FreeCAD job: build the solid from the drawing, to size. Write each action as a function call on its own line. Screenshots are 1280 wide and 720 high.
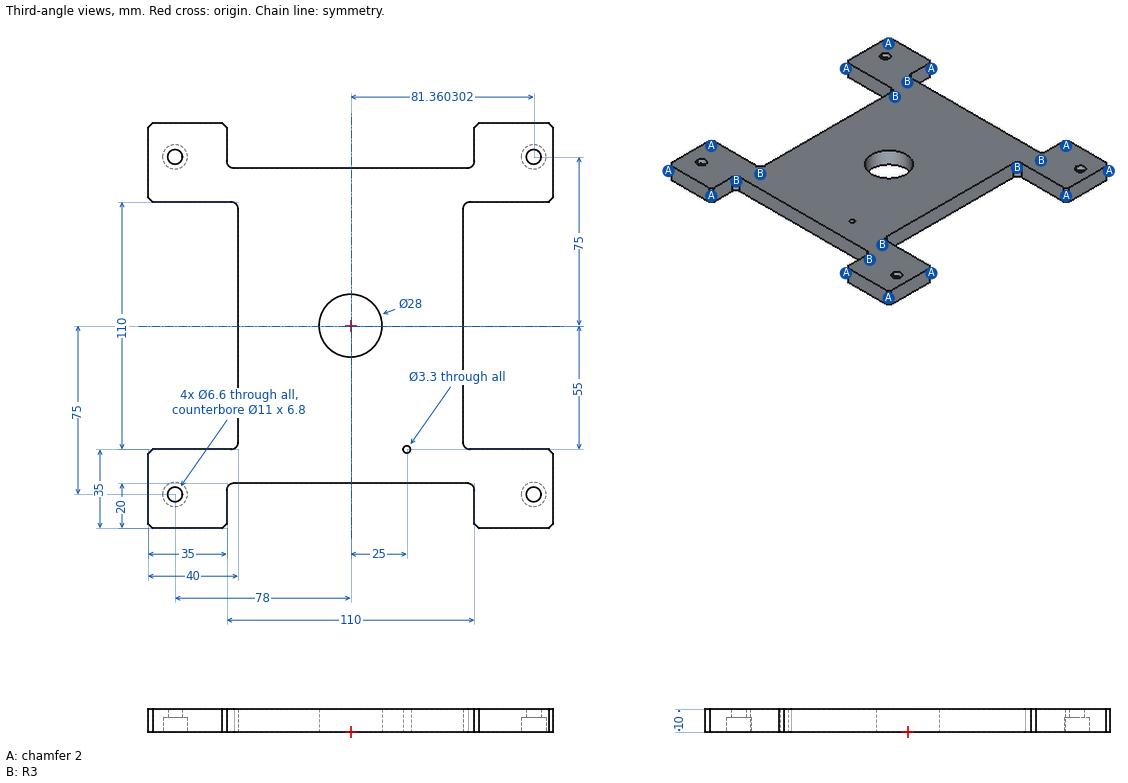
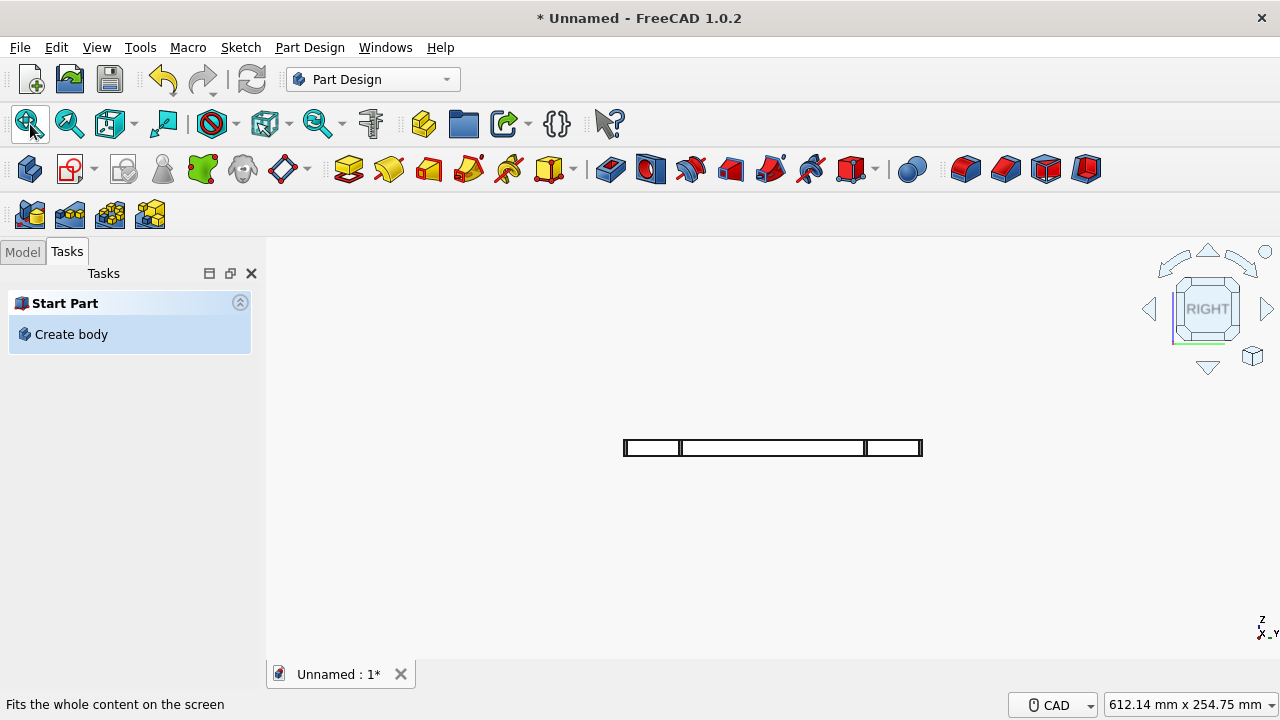
key(5)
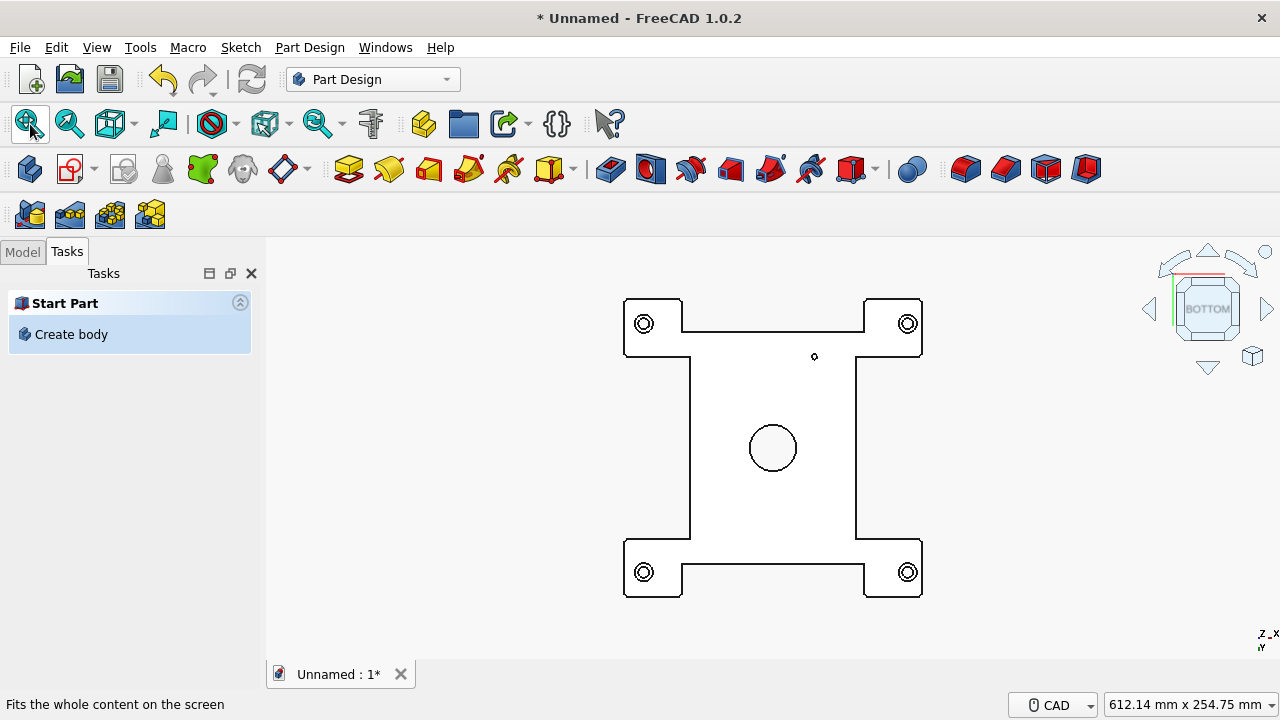
scroll(682, 563, up, 5)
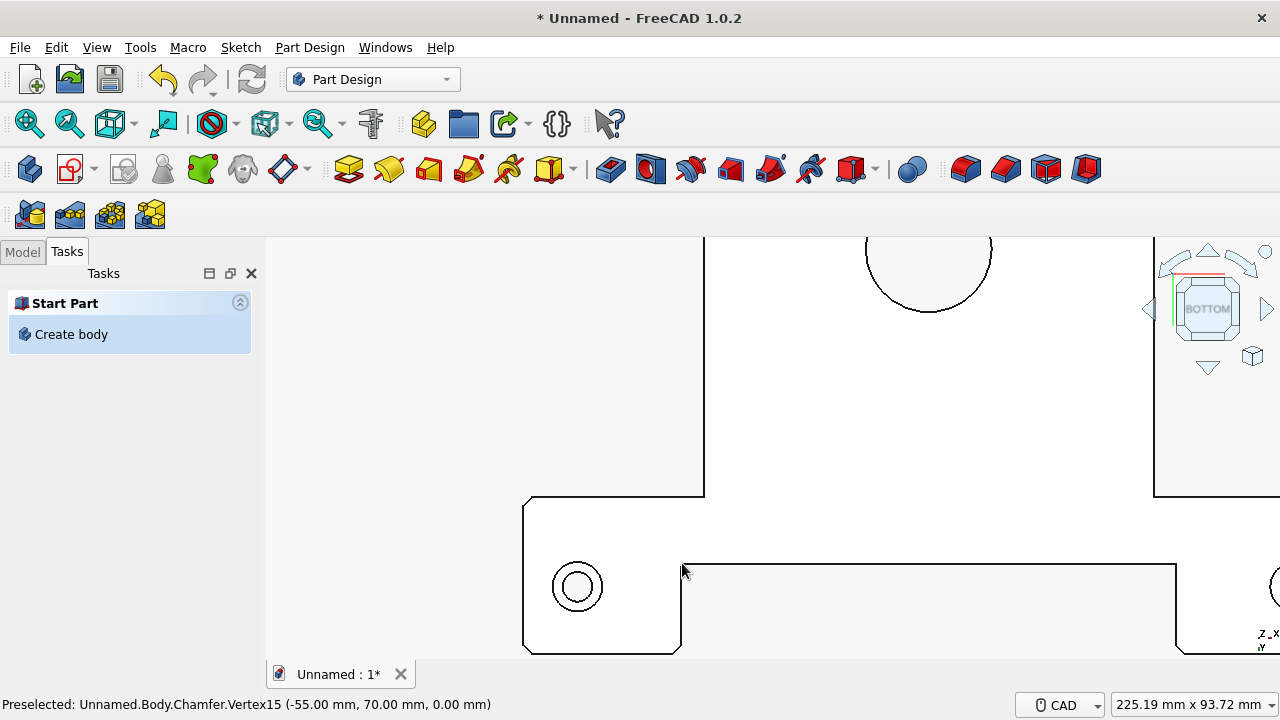
key(v)
key(f)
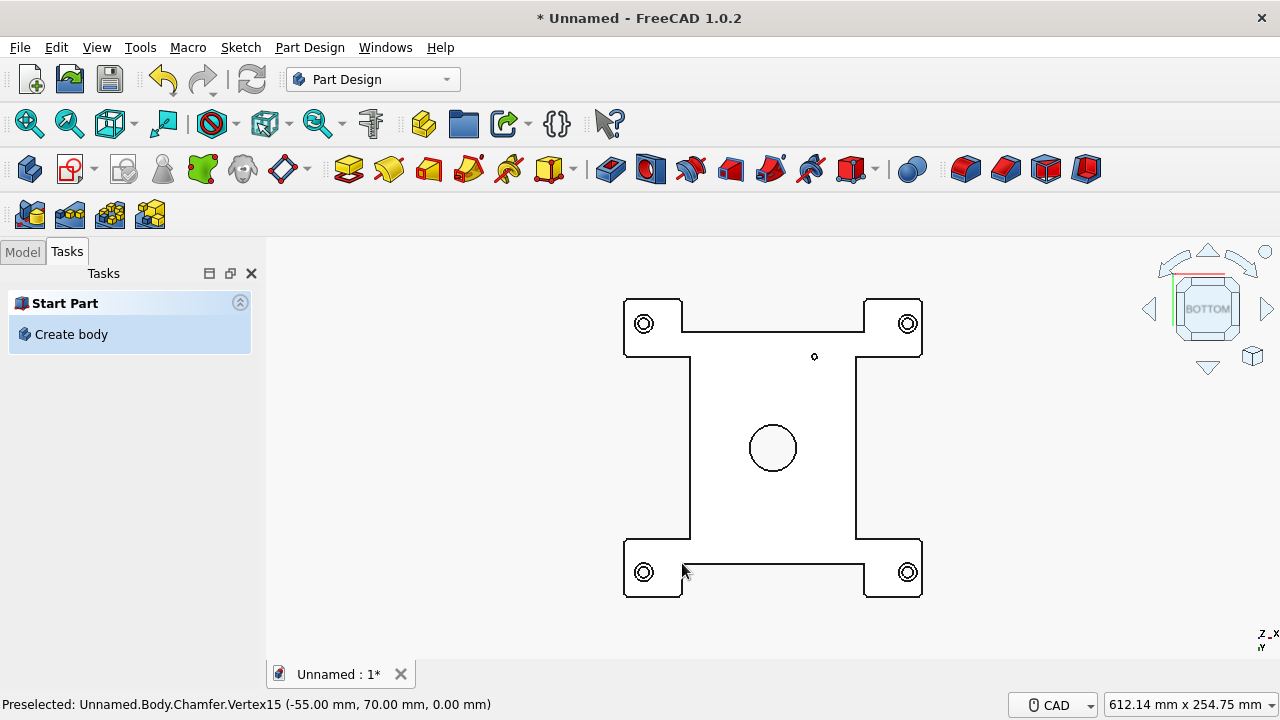
key(4)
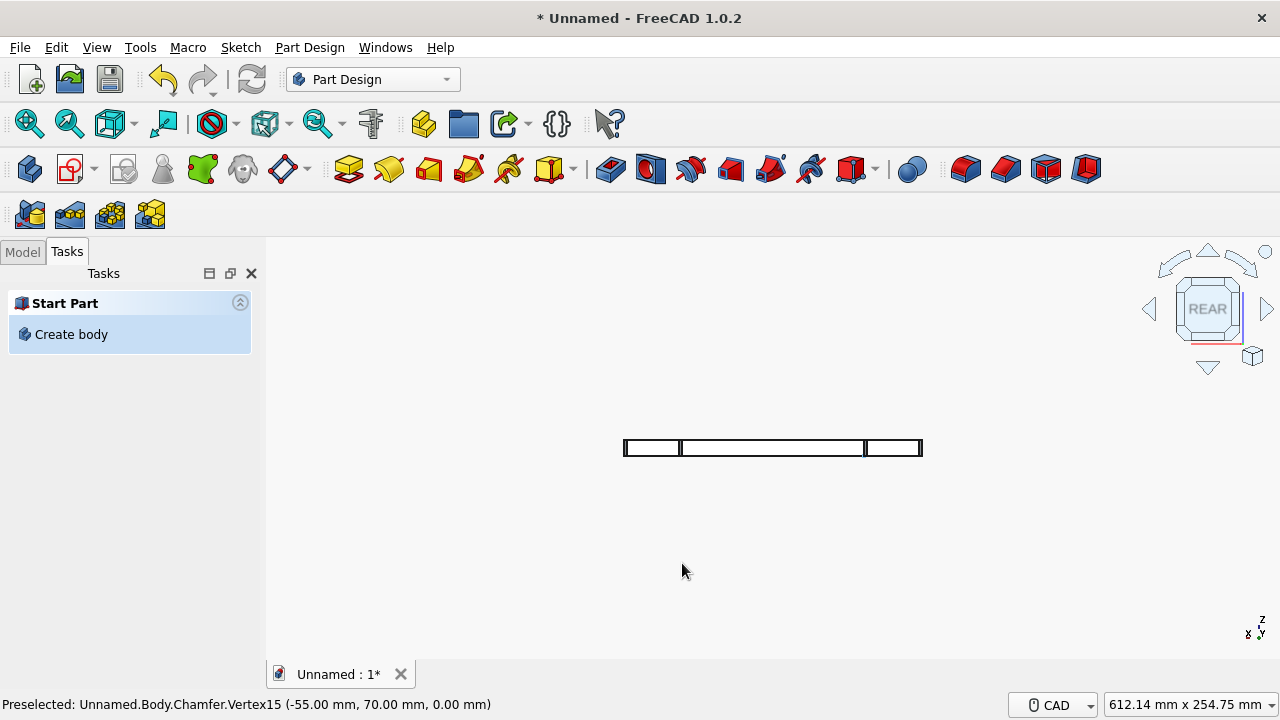
key(v)
key(f)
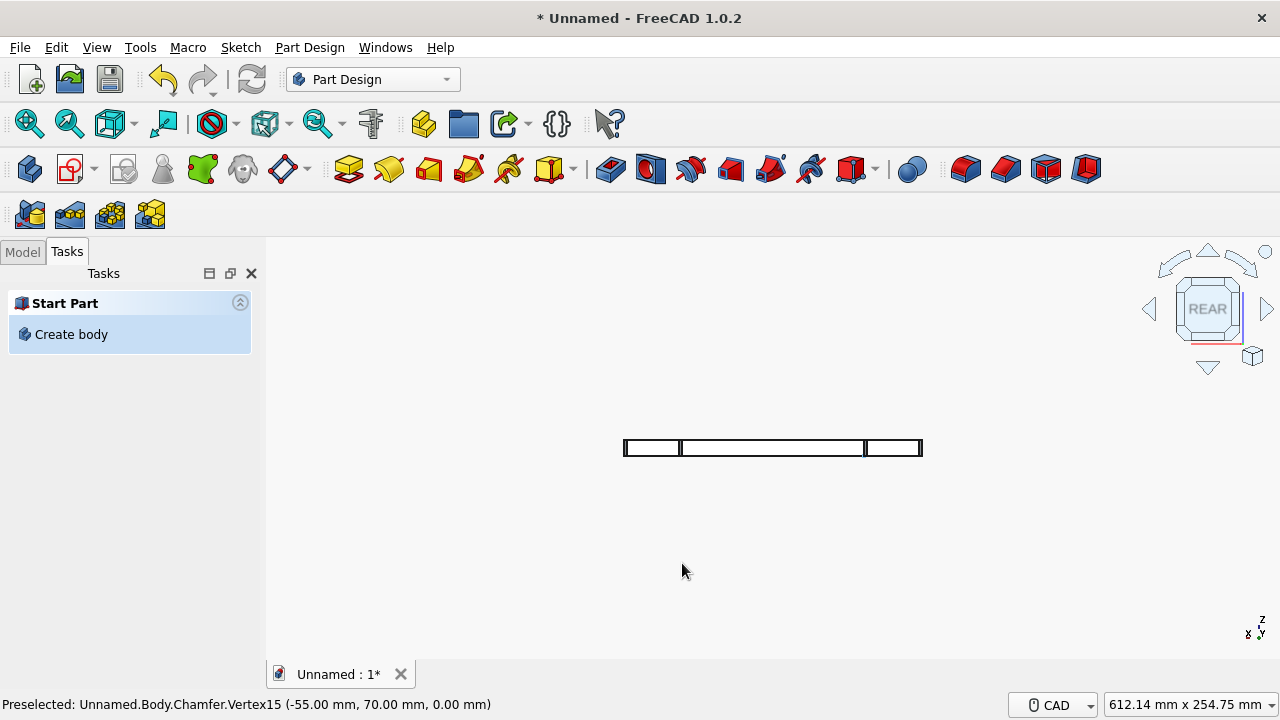
scroll(864, 447, up, 5)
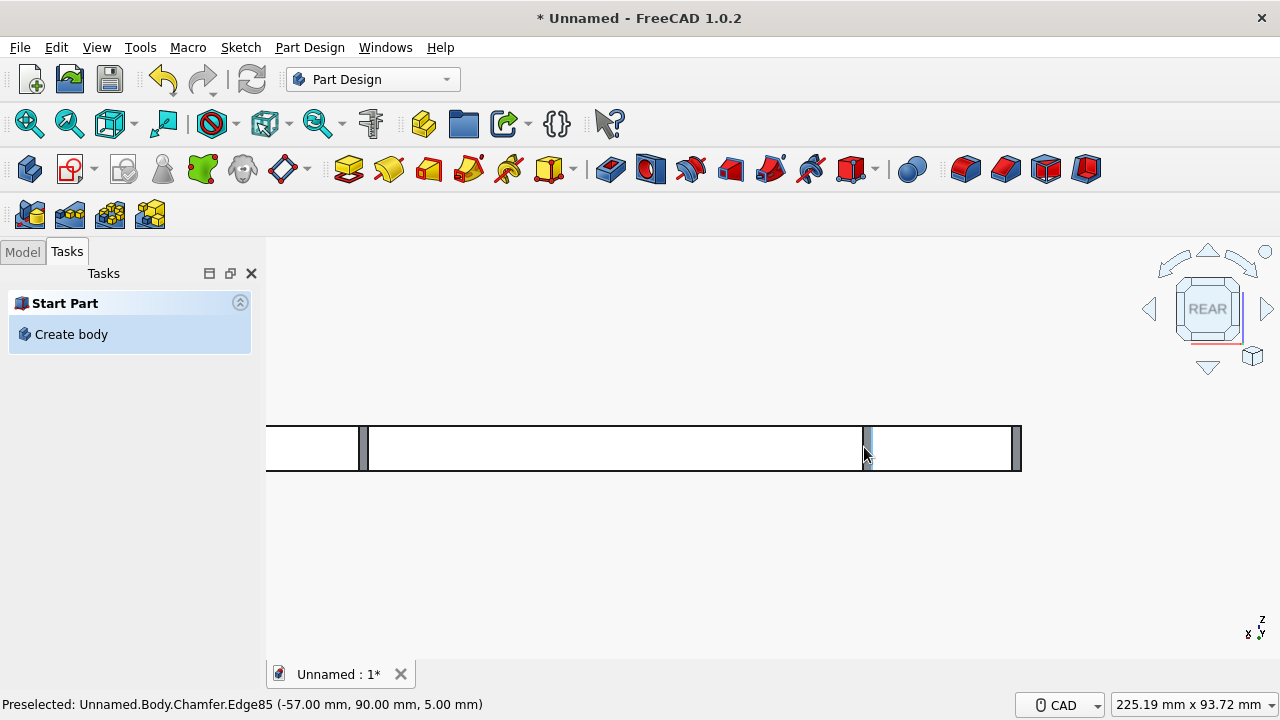
click(30, 124)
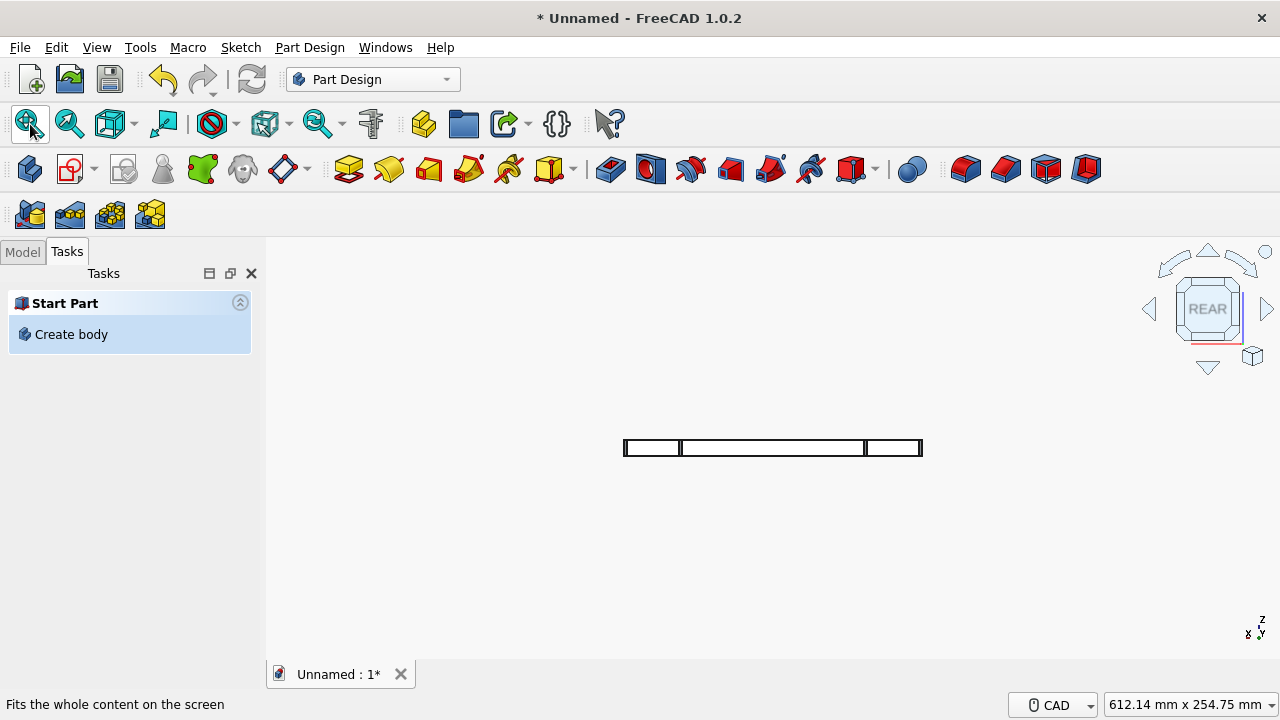
key(6)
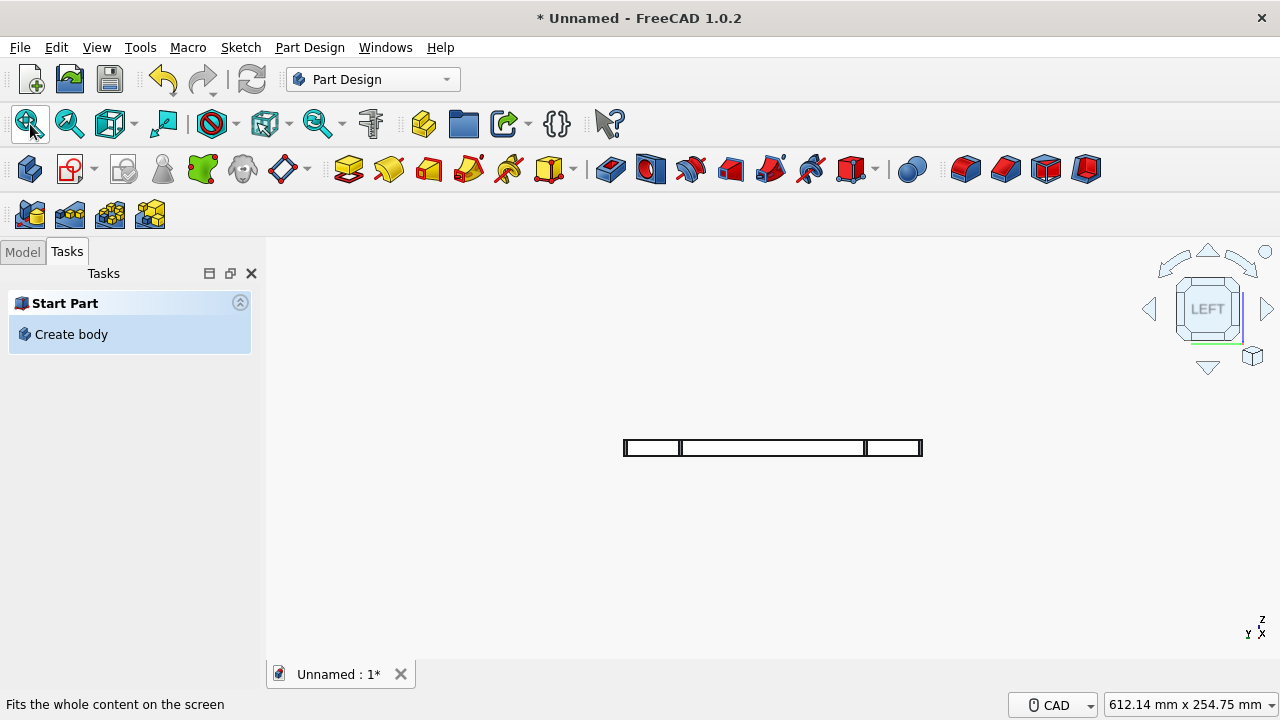
click(30, 124)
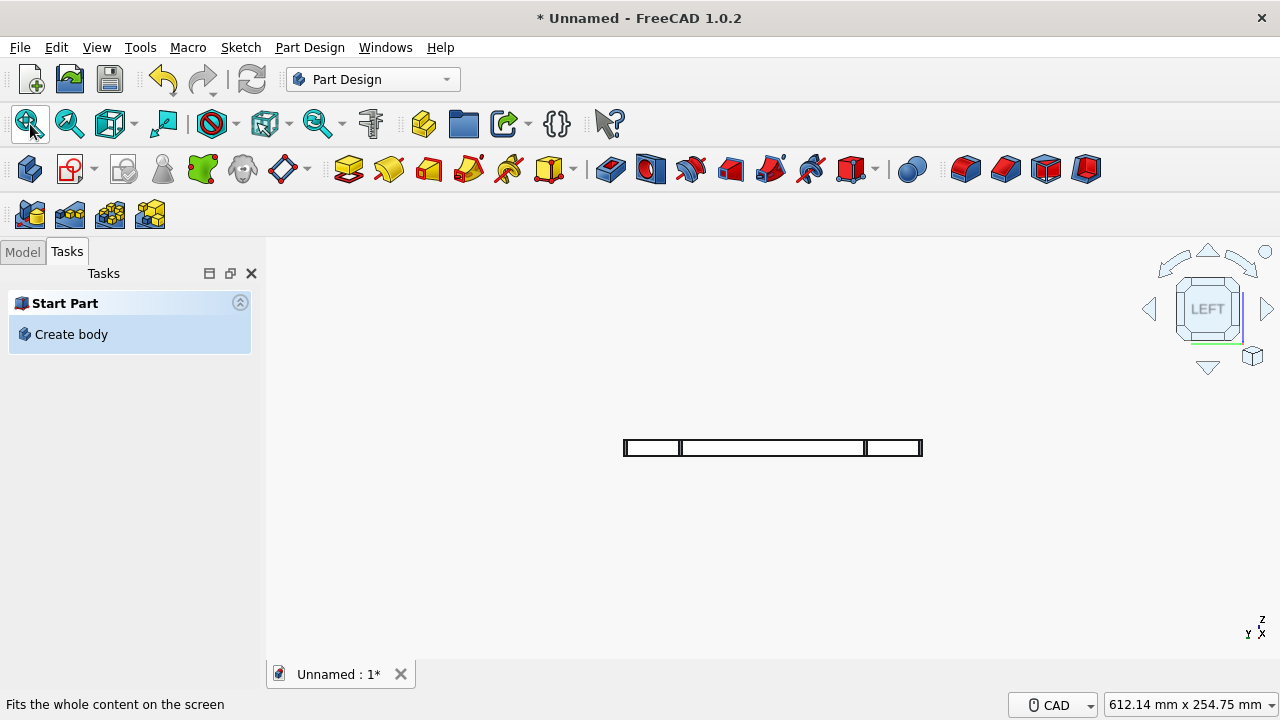
scroll(657, 447, up, 5)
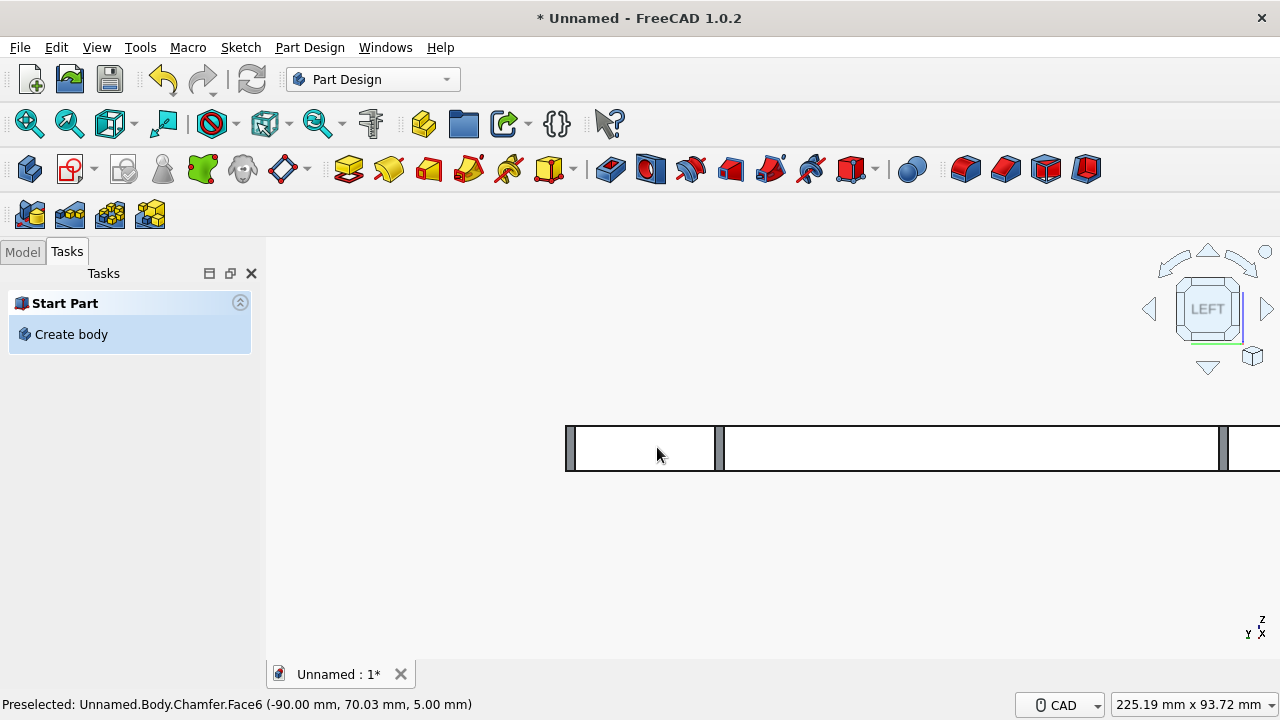
key(v)
key(f)